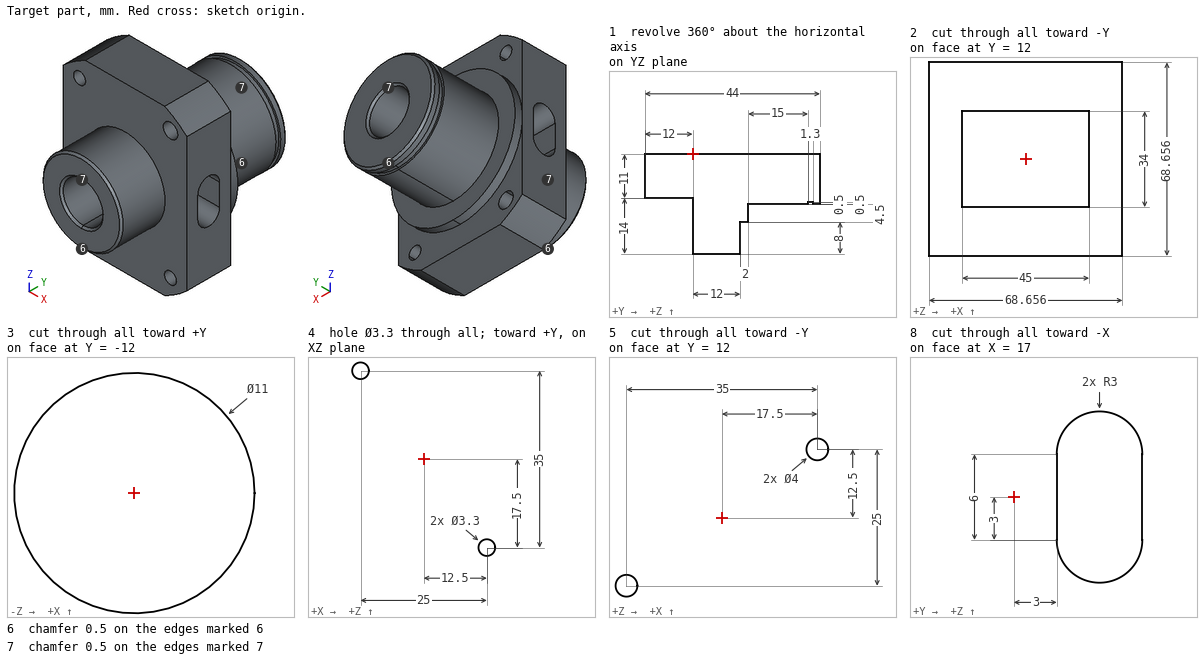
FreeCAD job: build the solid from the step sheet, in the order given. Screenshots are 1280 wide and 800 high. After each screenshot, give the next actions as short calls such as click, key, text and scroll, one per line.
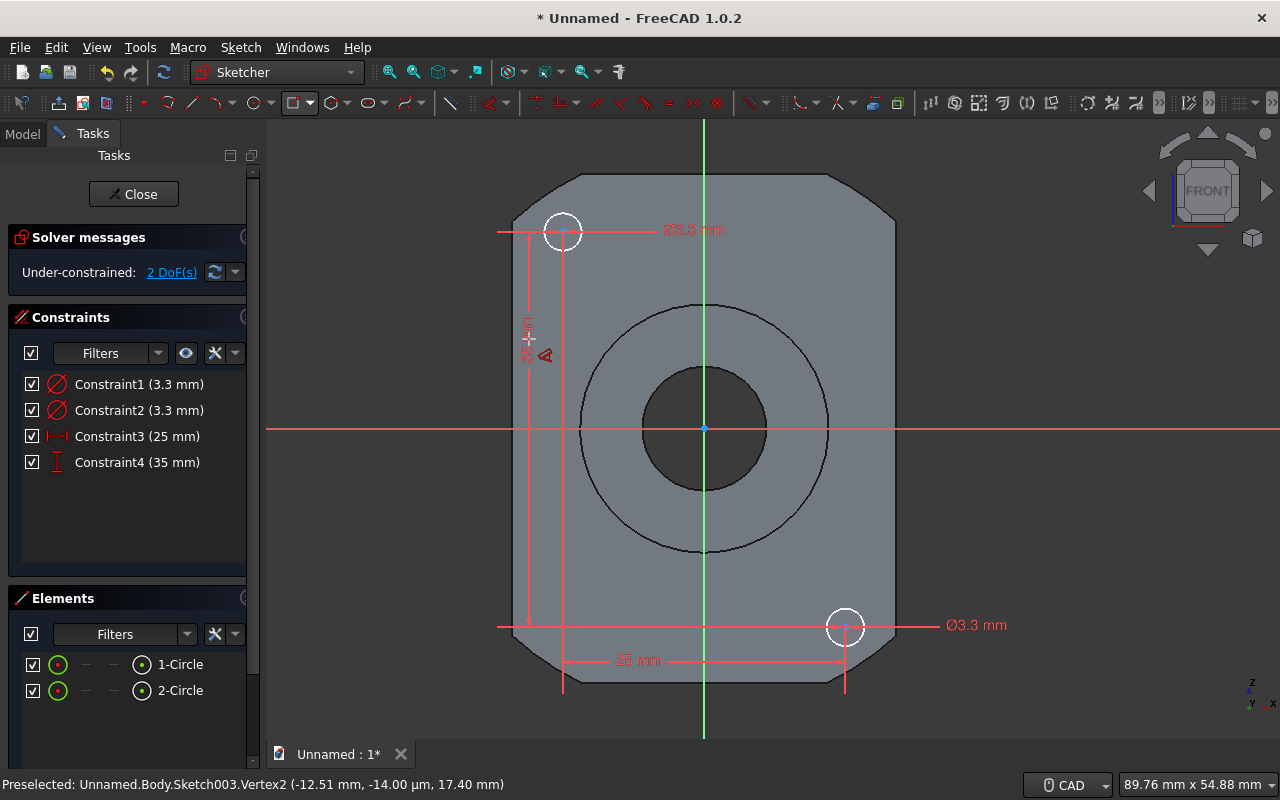
click(845, 627)
click(775, 661)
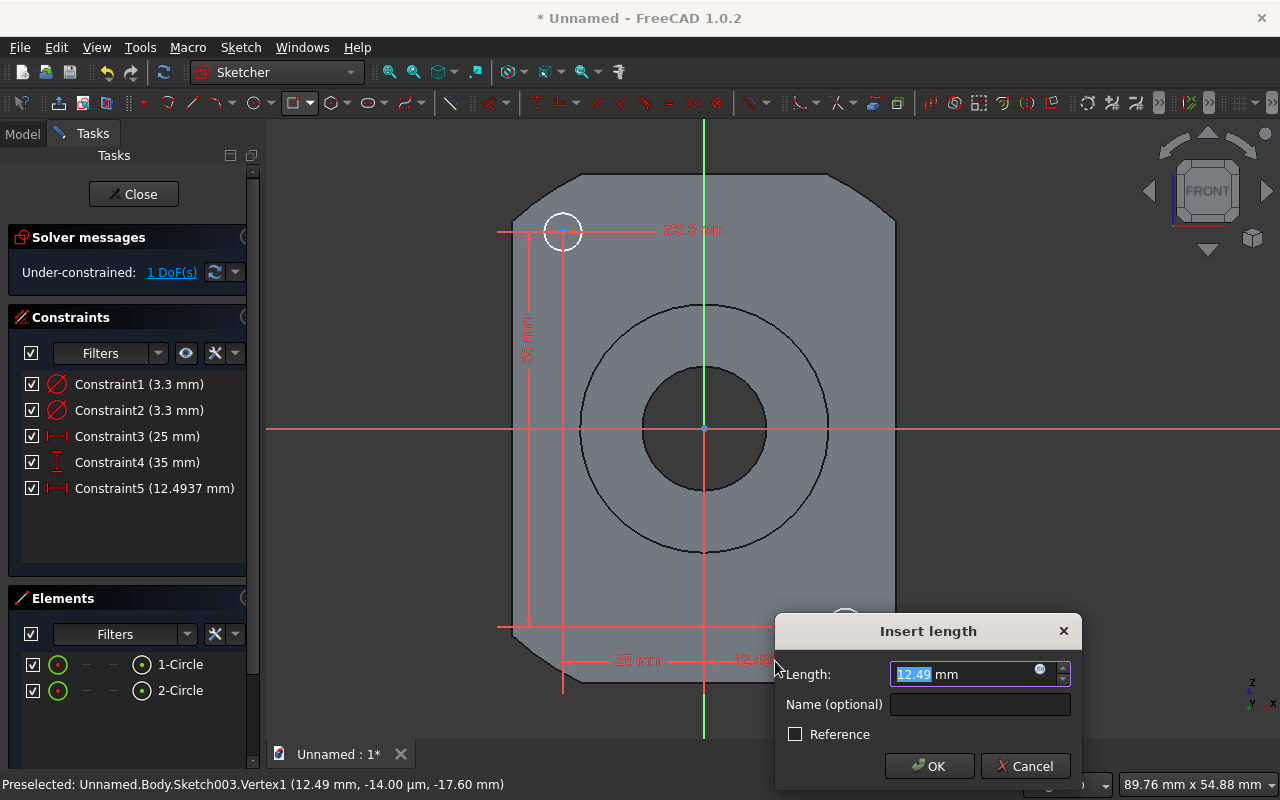
text(12.5)
key(Return)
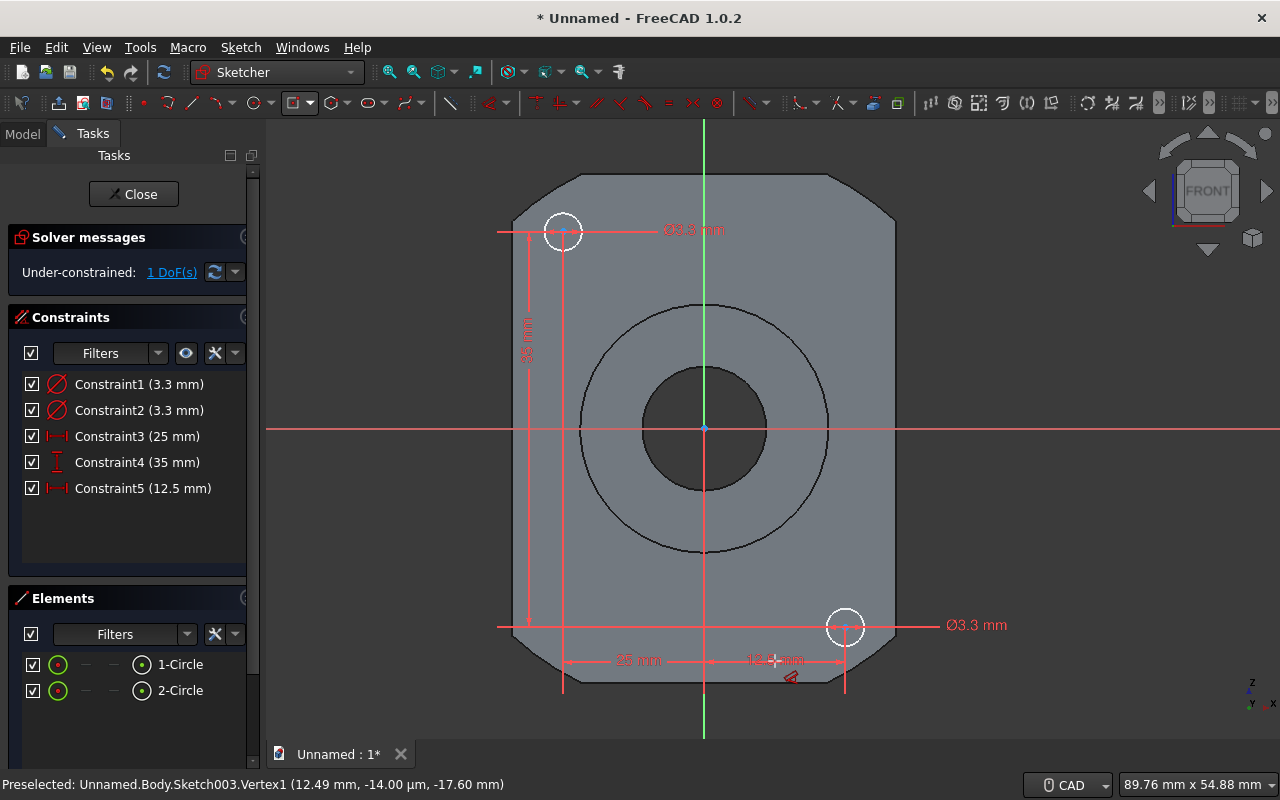
click(845, 627)
click(879, 528)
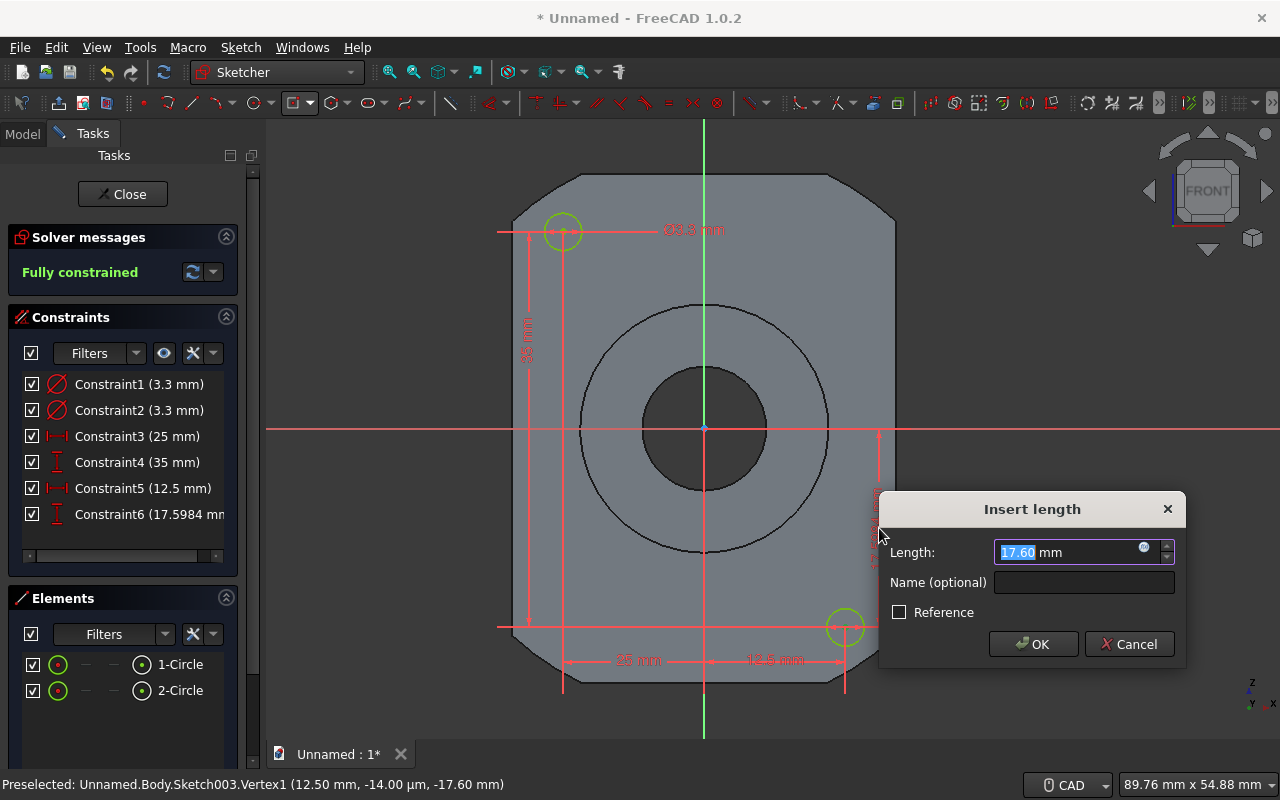
text(17.5)
key(Return)
key(Escape)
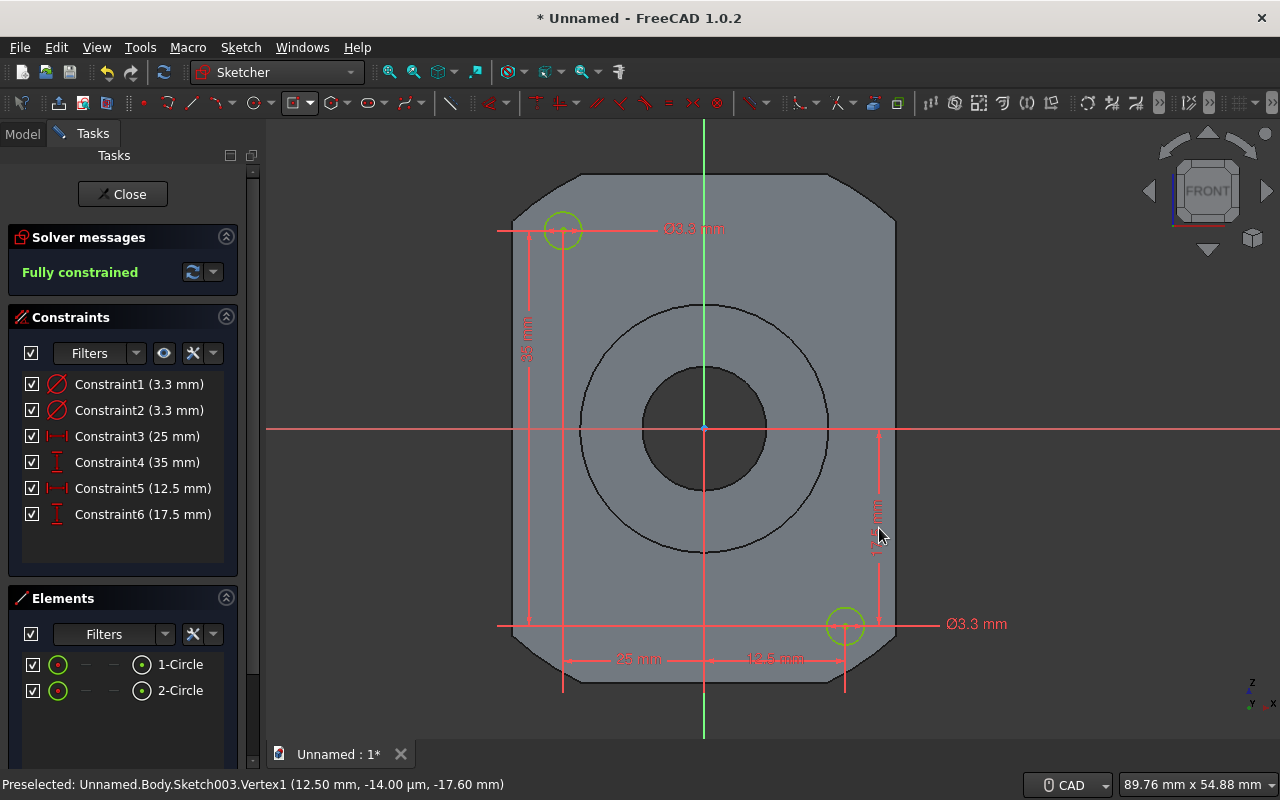
click(123, 194)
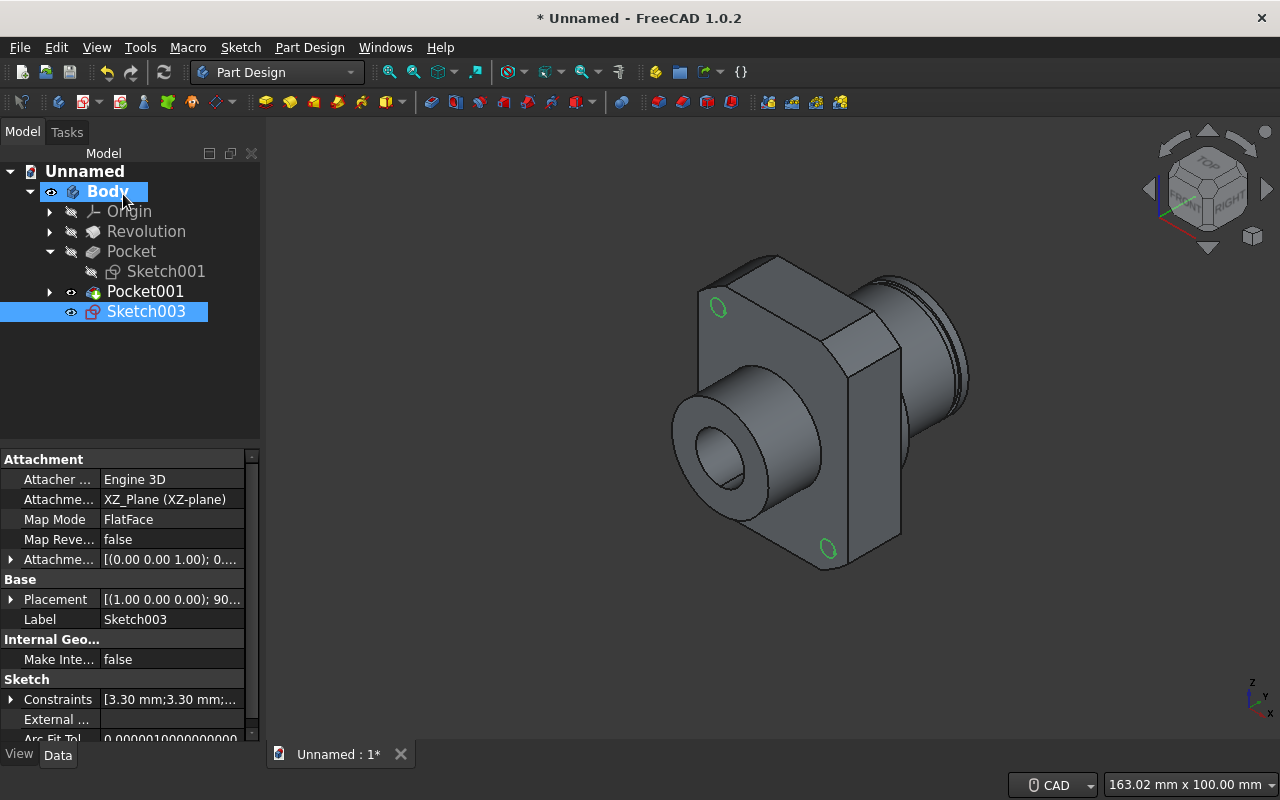
click(456, 102)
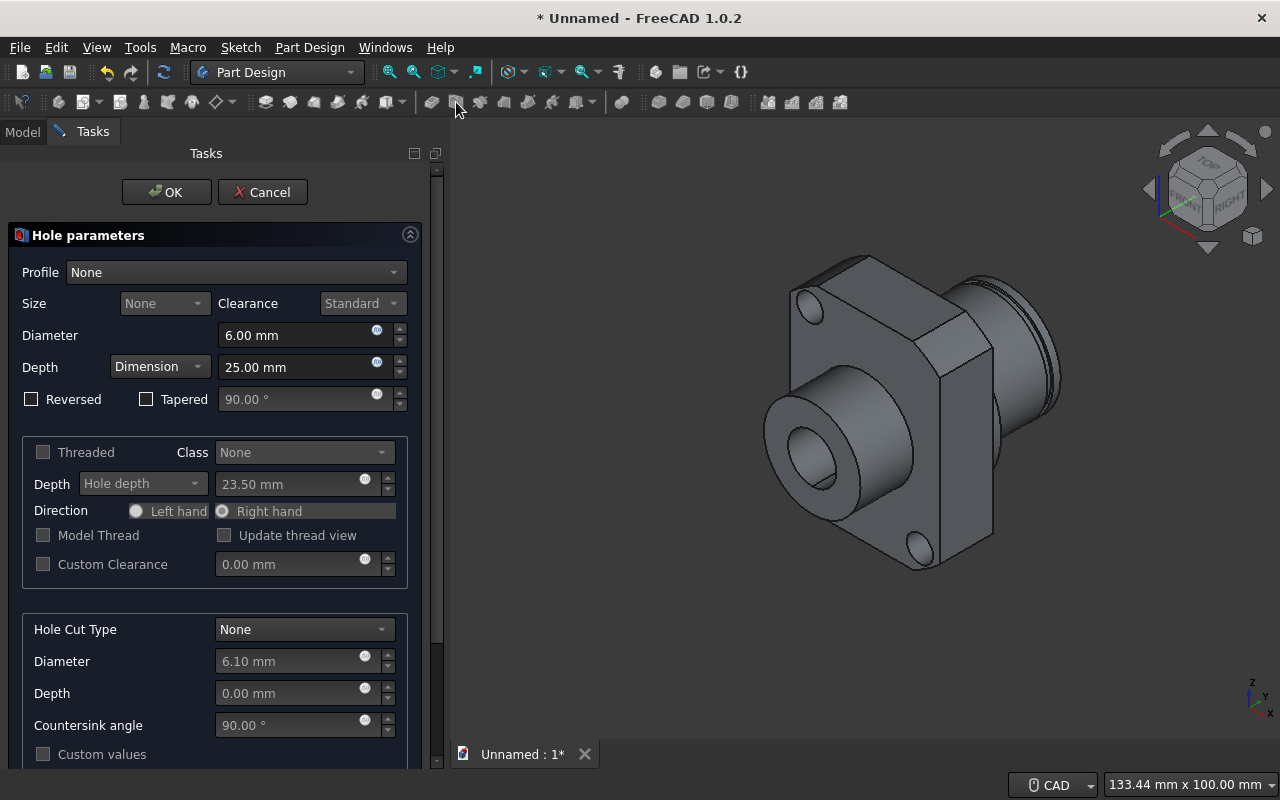
triple_click(305, 335)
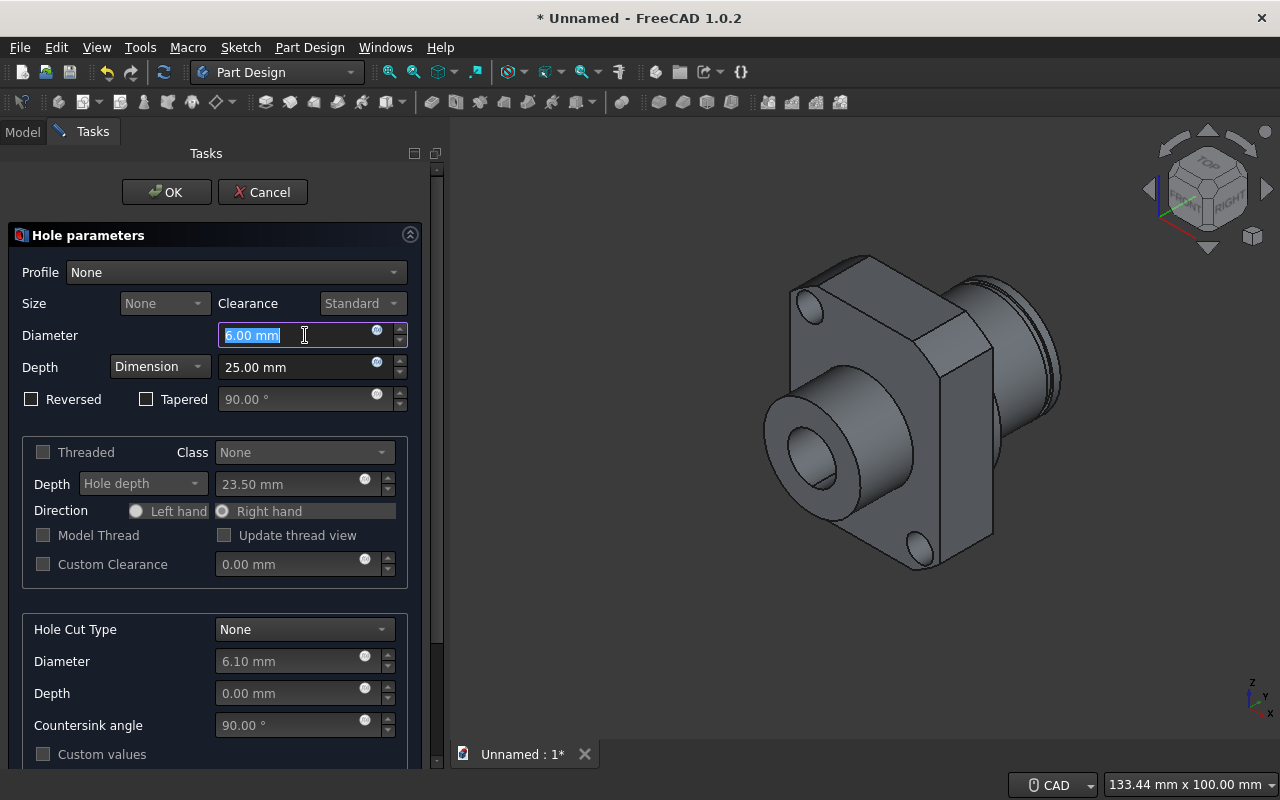
text(3.3)
key(Tab)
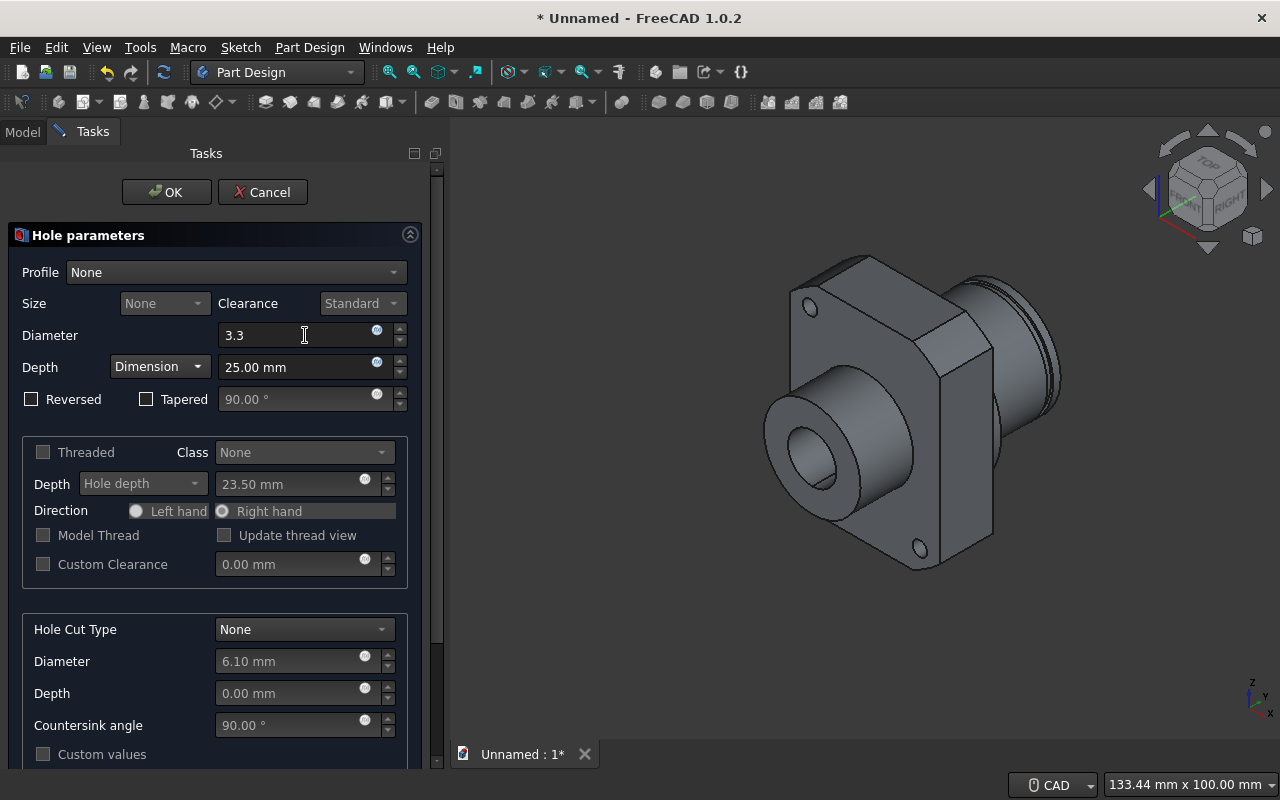
click(161, 366)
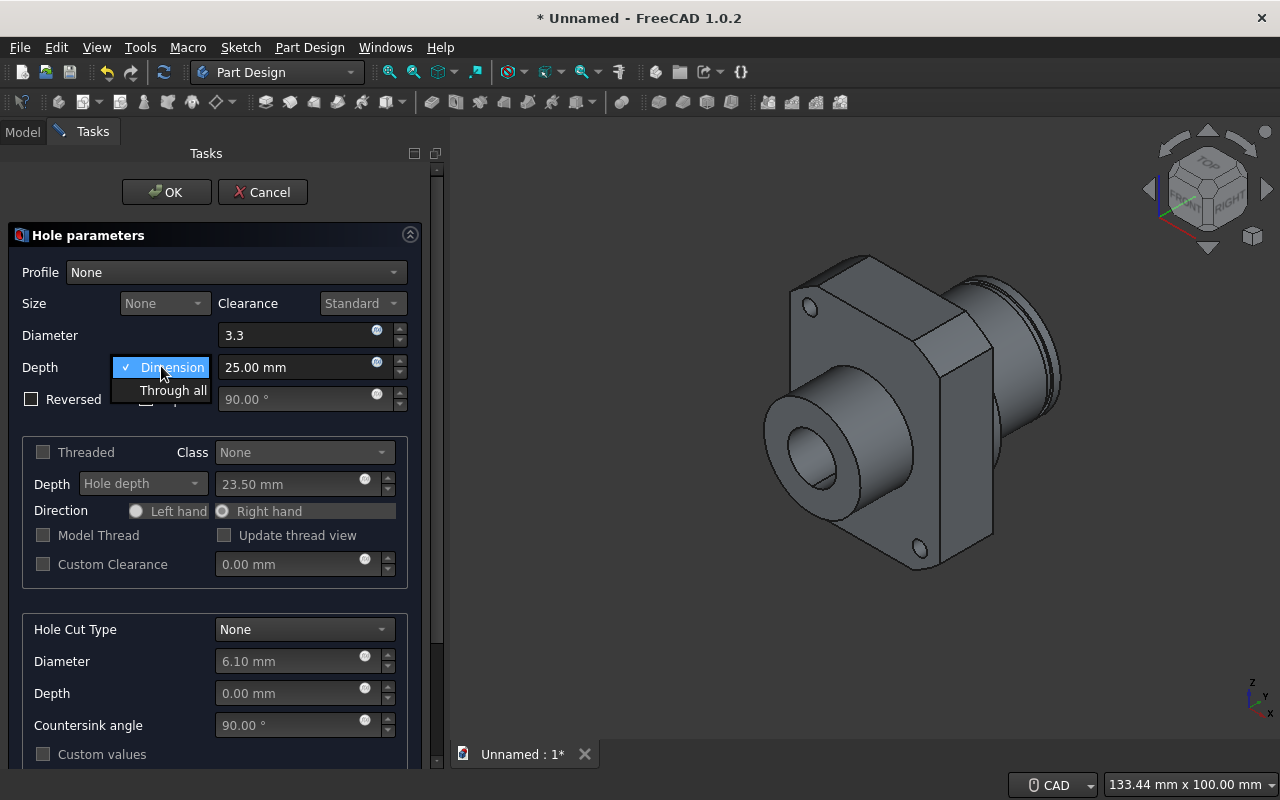
click(160, 390)